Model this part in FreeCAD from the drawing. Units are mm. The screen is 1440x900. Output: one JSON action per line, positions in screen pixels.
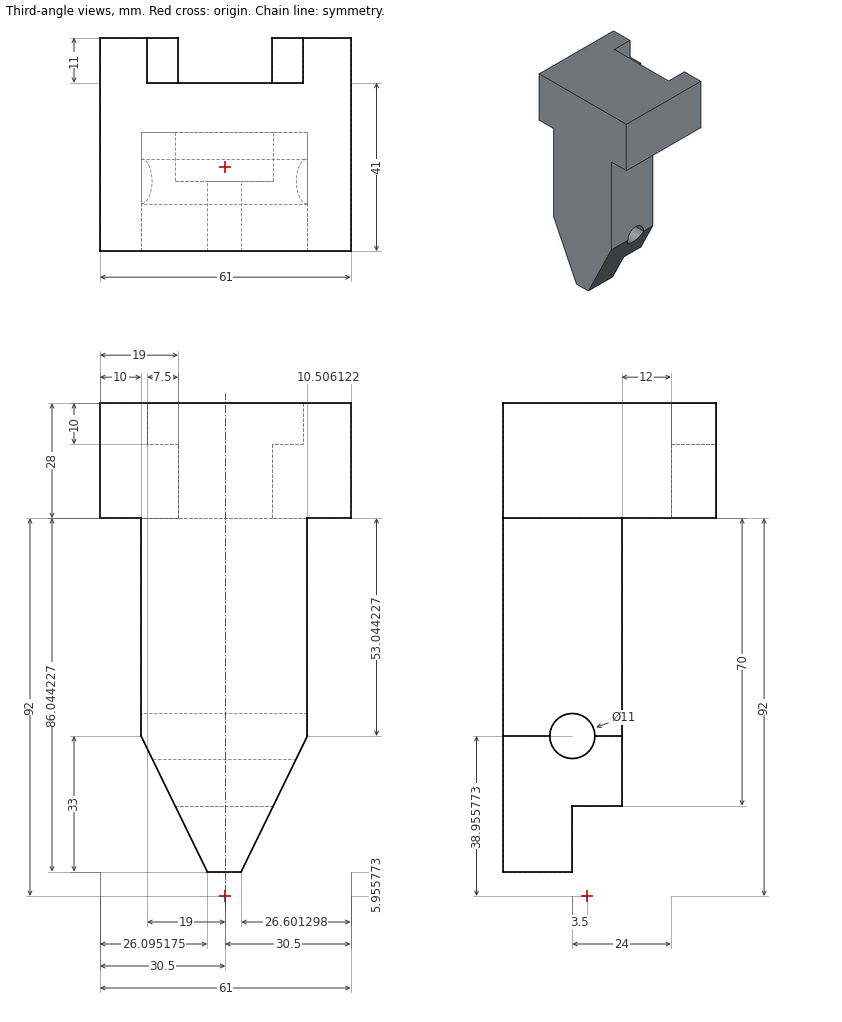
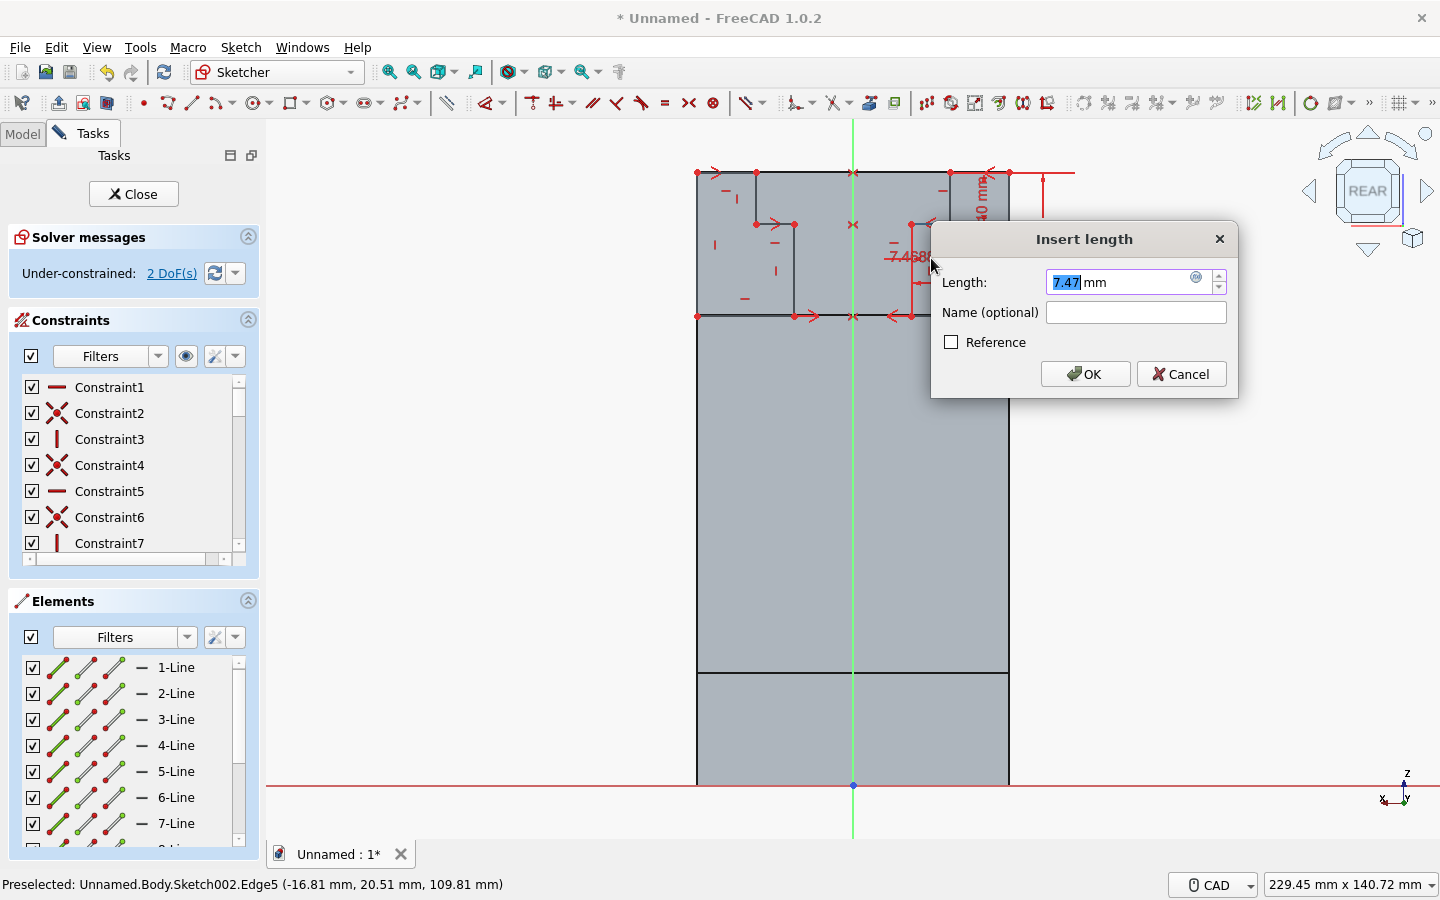
{"action": "type", "text": "7.5"}
{"action": "key", "text": "Return"}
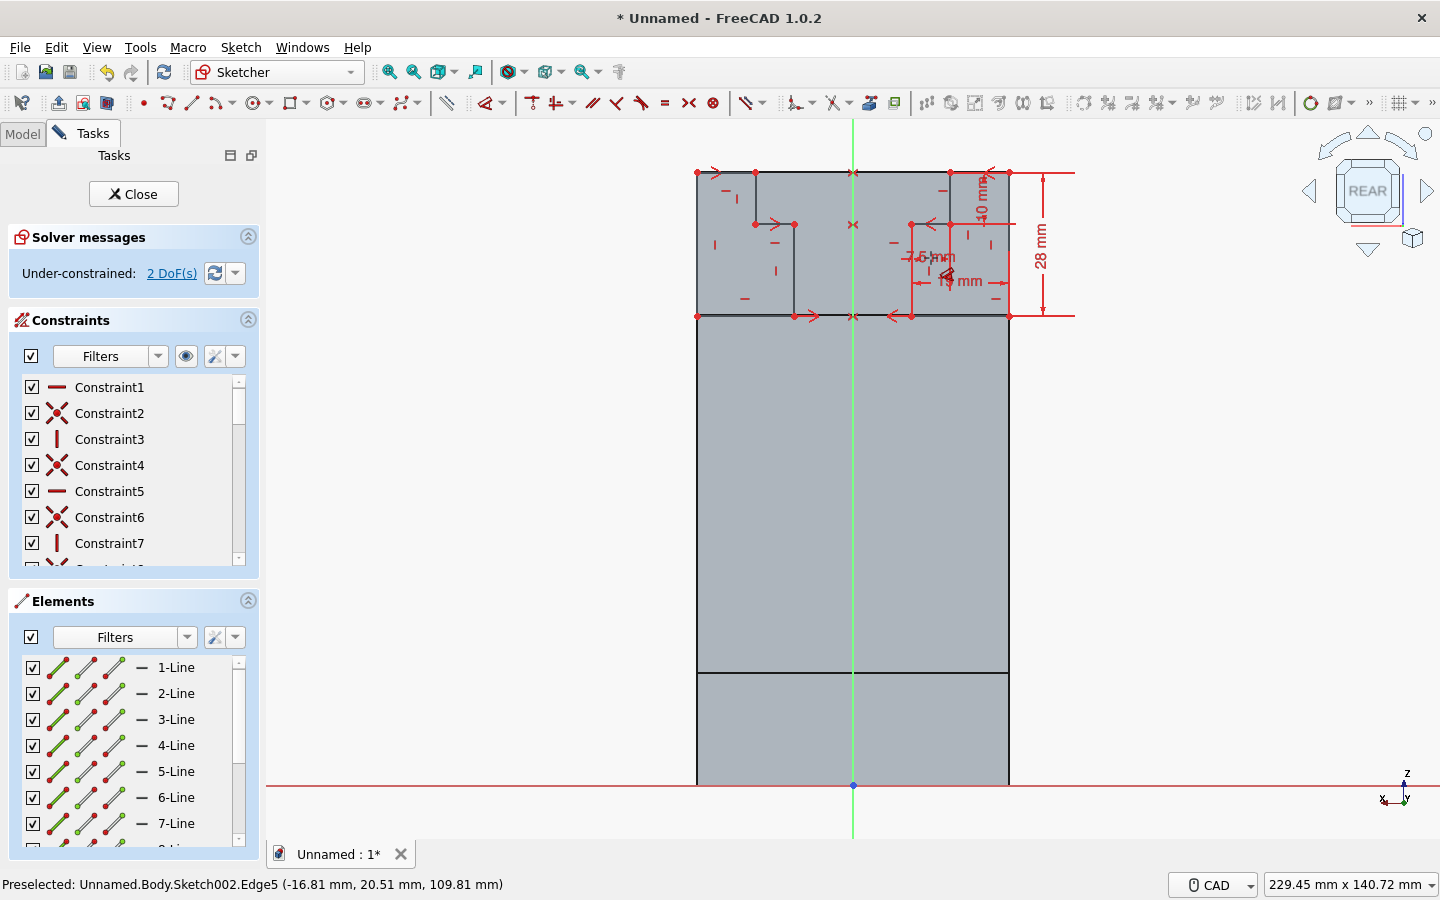
{"action": "left_click", "coordinate": [912, 316]}
{"action": "left_click", "coordinate": [946, 551]}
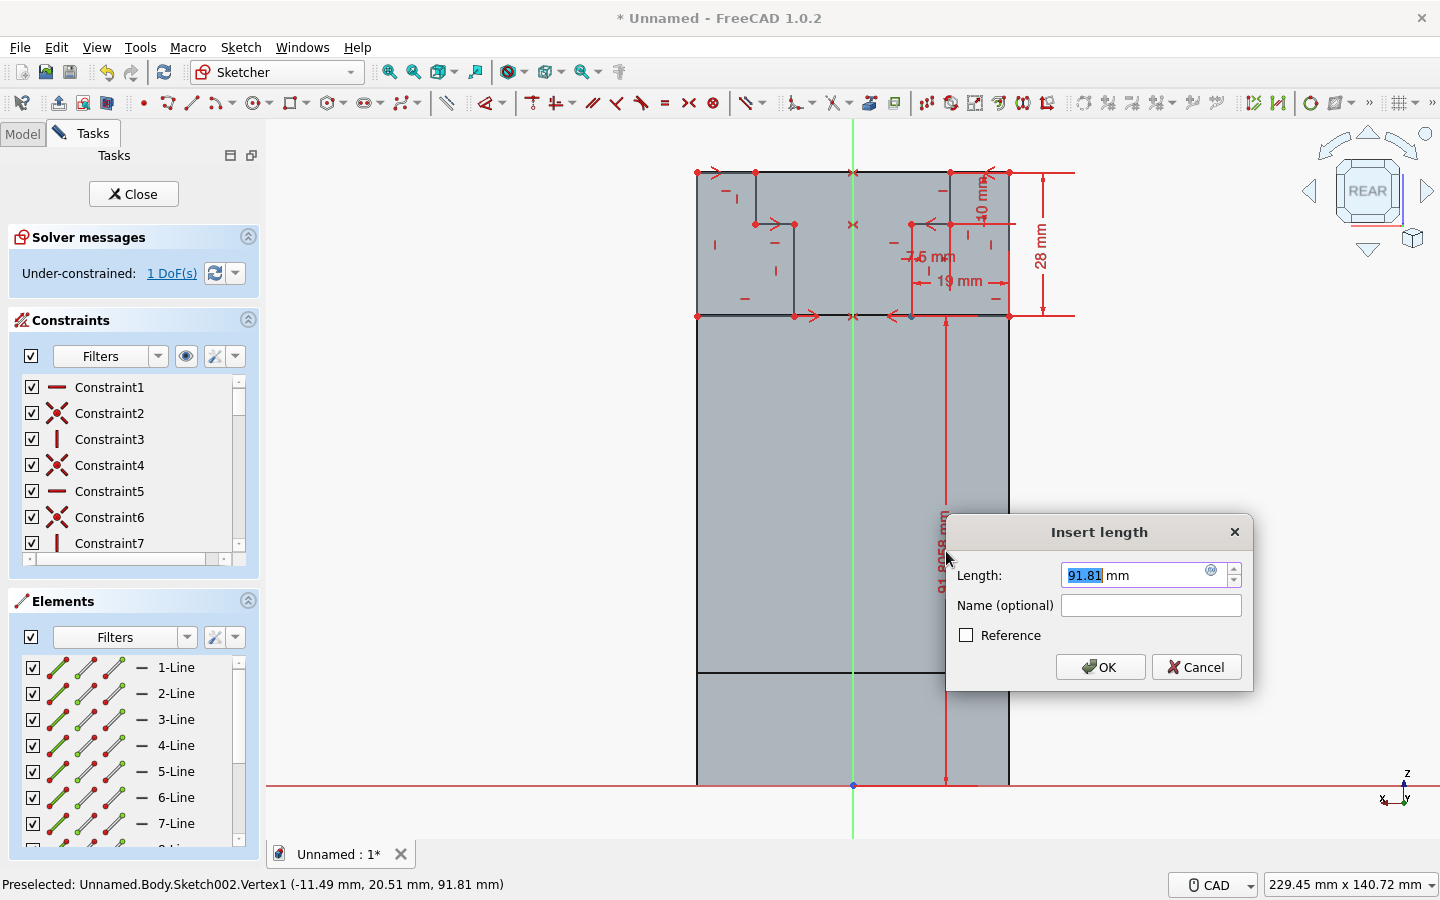
{"action": "type", "text": "92"}
{"action": "key", "text": "Return"}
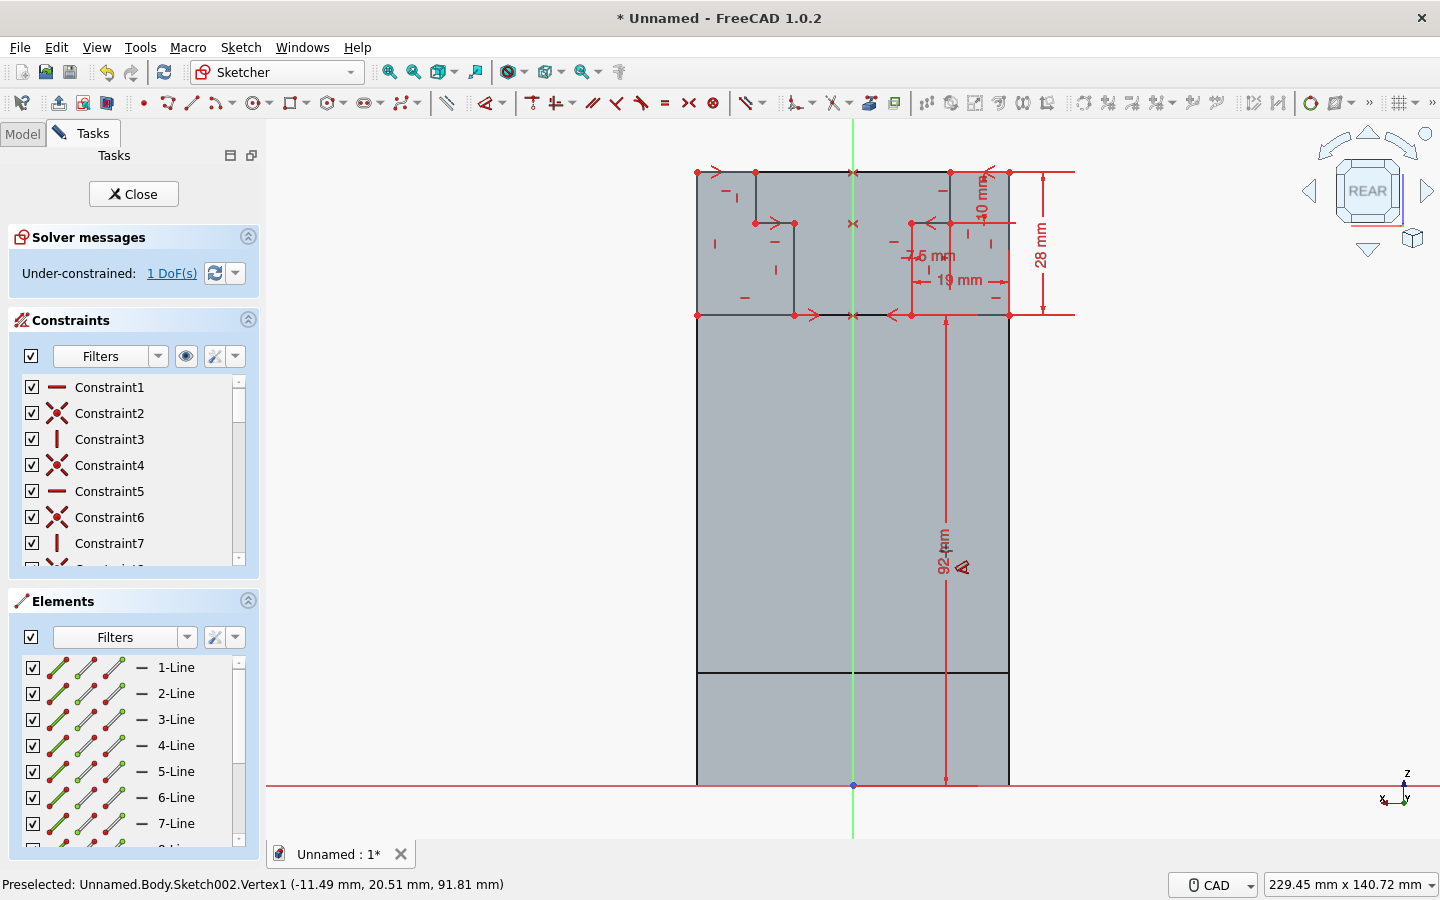
{"action": "left_click", "coordinate": [950, 172]}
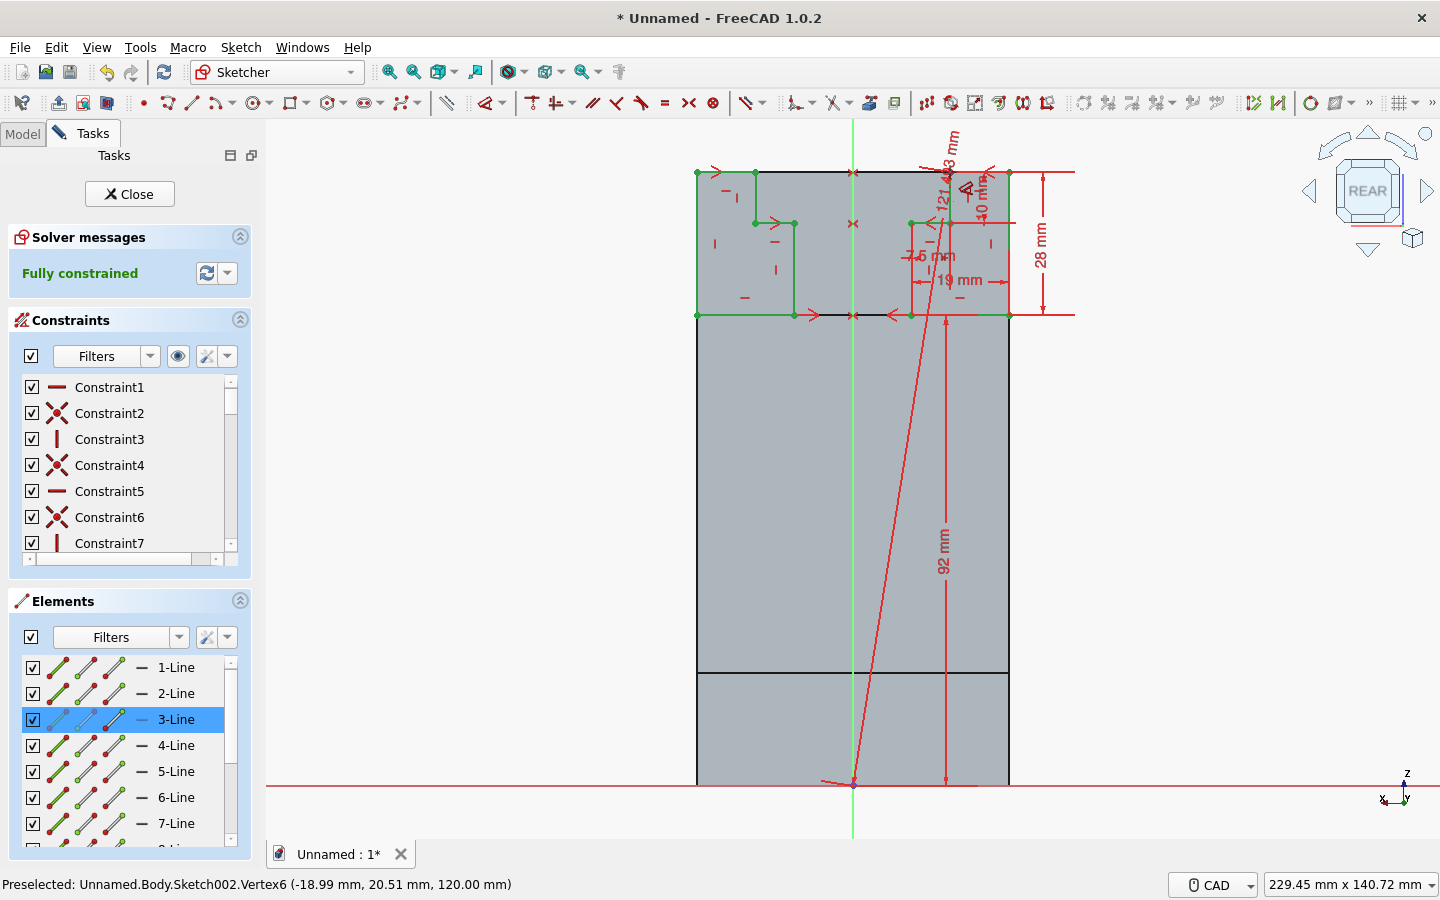
{"action": "key", "text": "Escape"}
{"action": "key", "text": "Escape"}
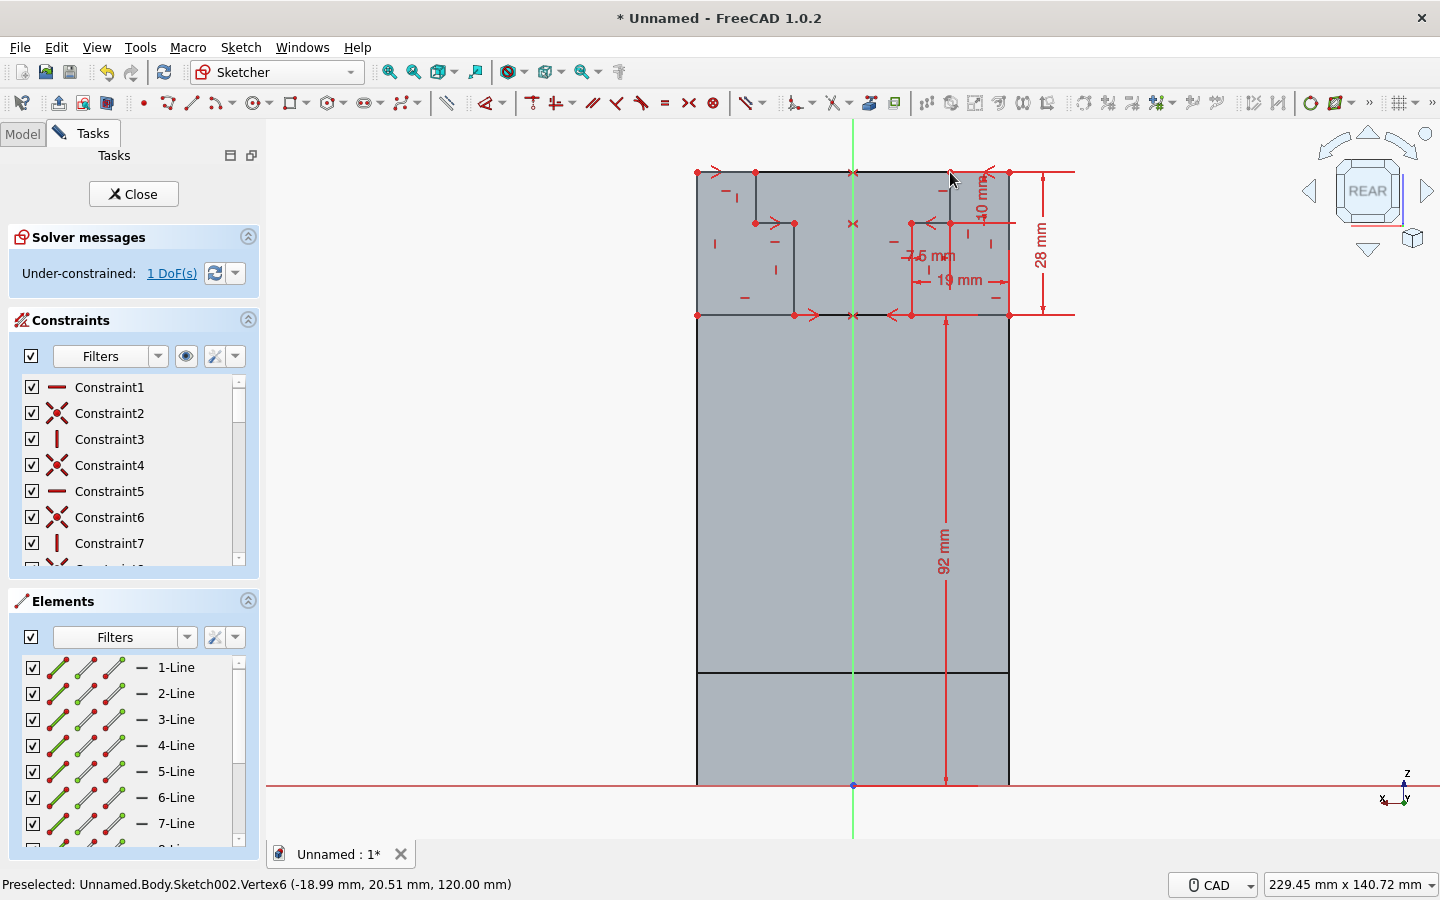
{"action": "left_click", "coordinate": [950, 172]}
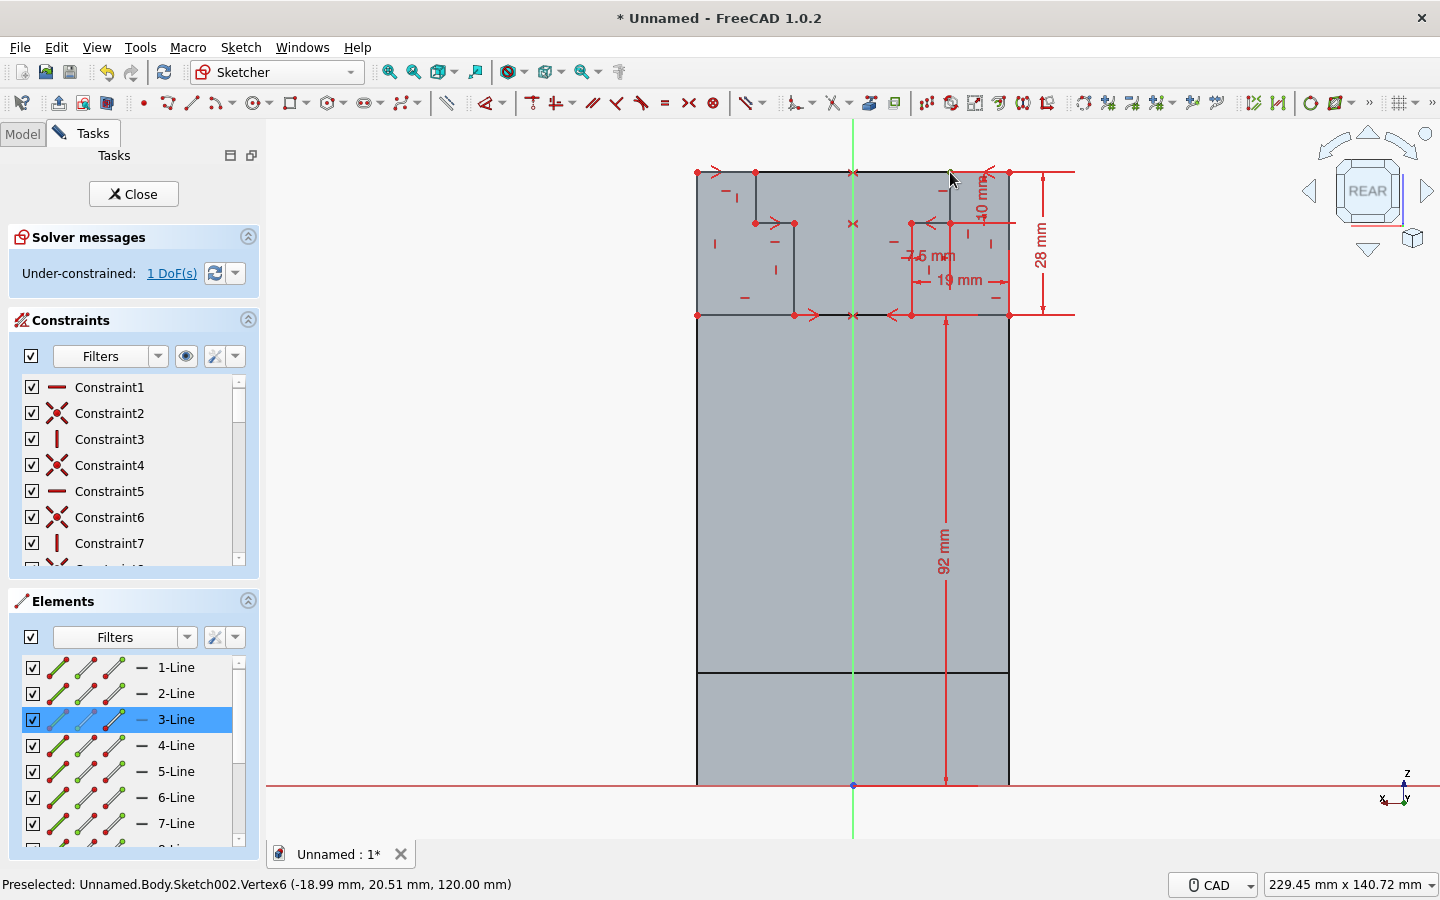
{"action": "left_click", "coordinate": [504, 104]}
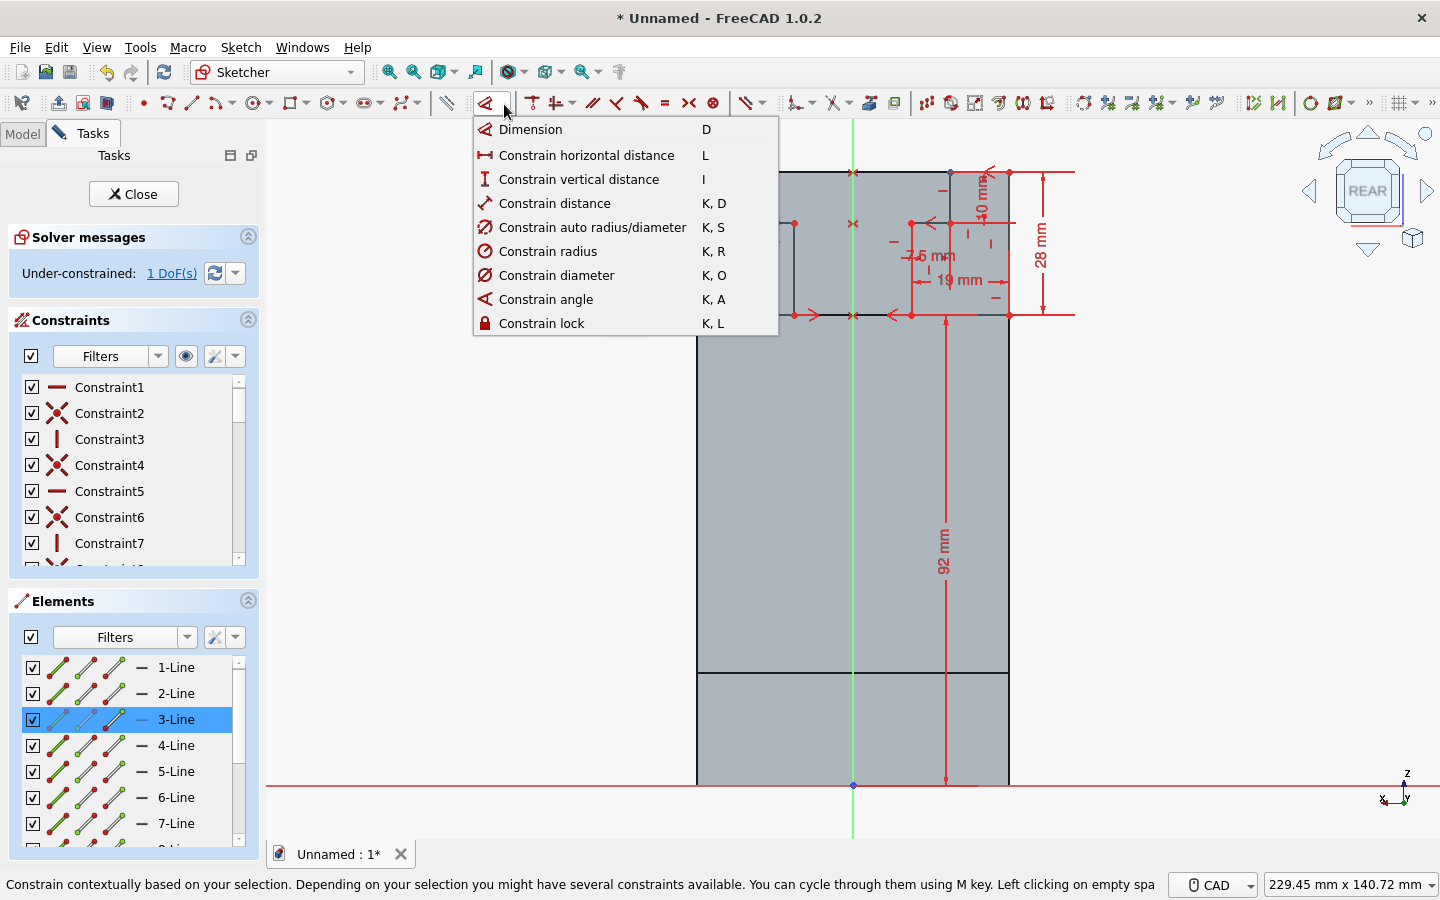
{"action": "left_click", "coordinate": [626, 155]}